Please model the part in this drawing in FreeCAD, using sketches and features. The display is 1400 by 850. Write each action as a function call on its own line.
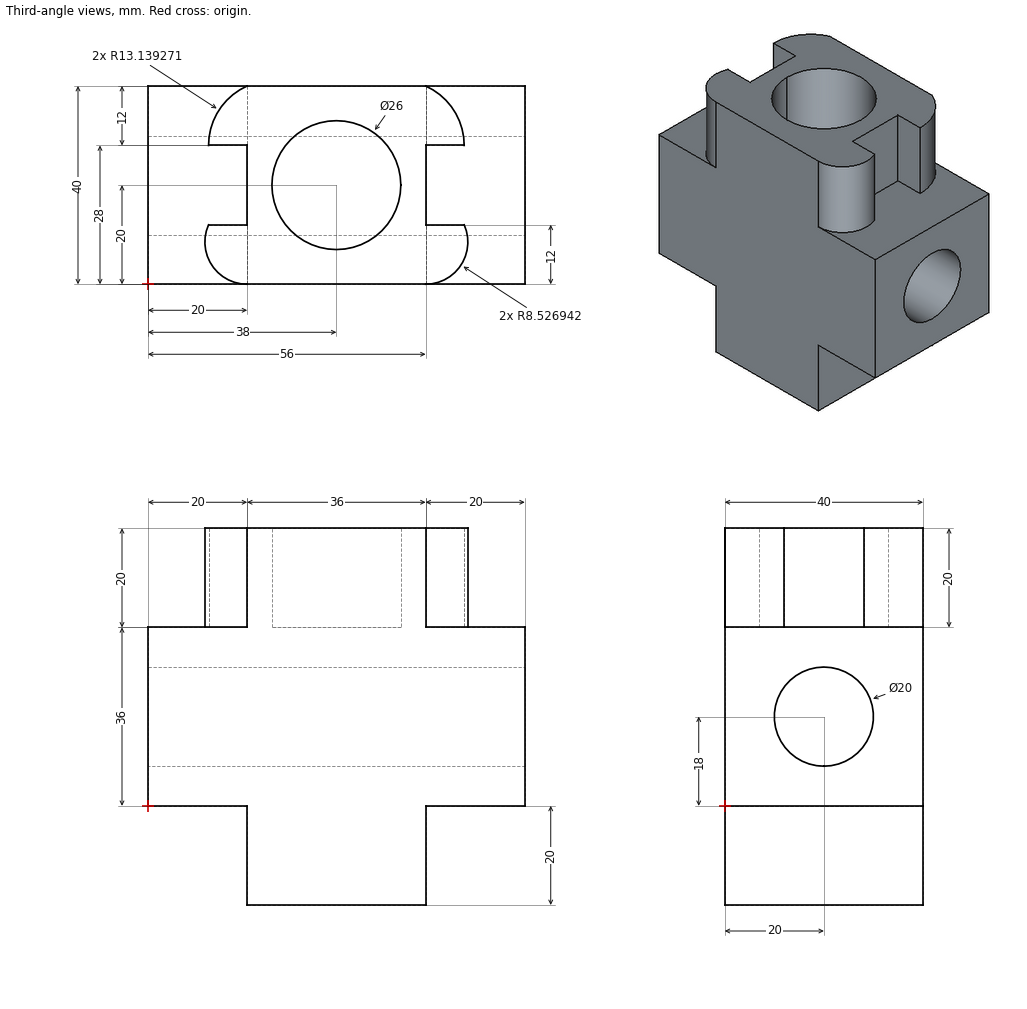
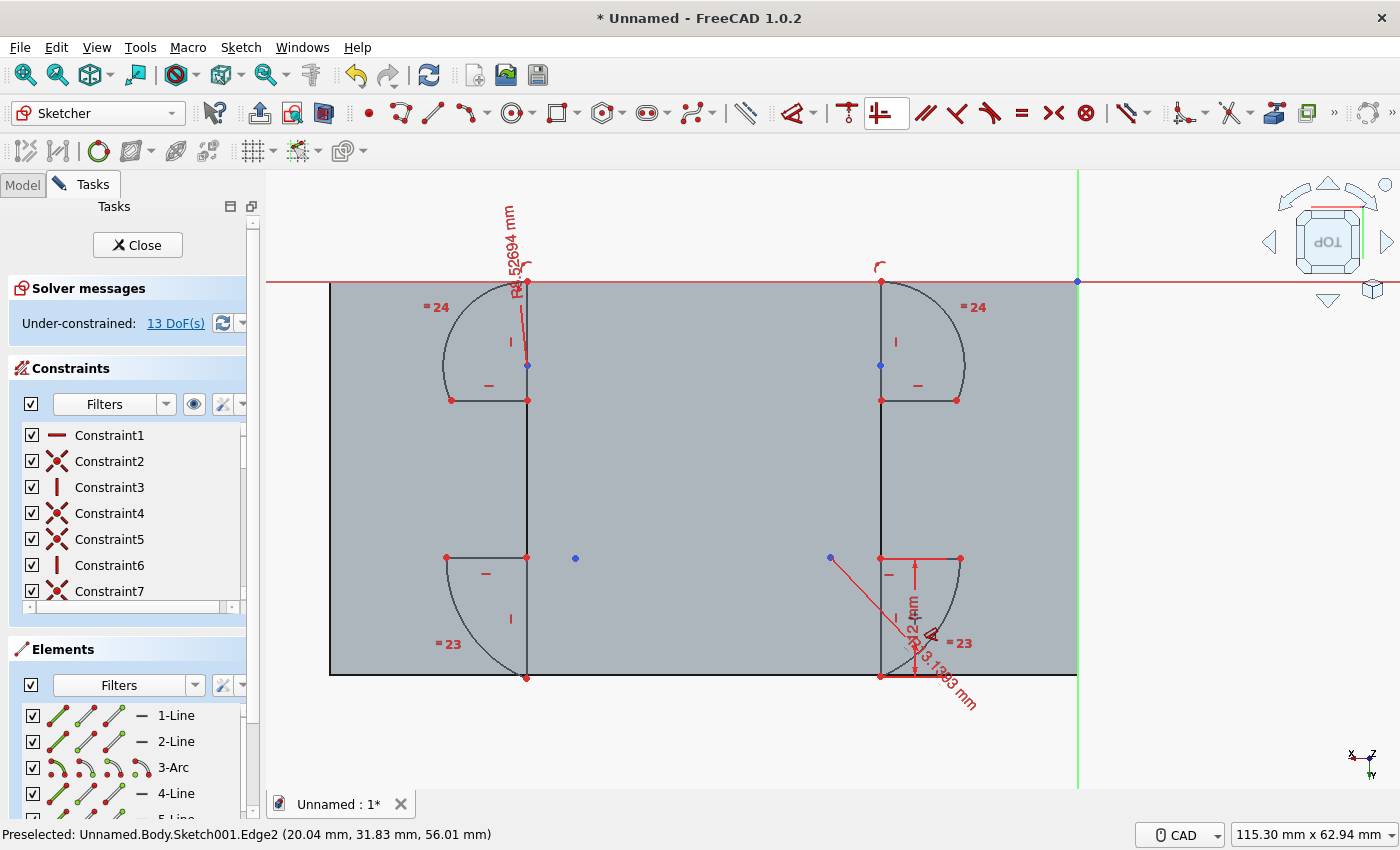
click(527, 642)
click(493, 618)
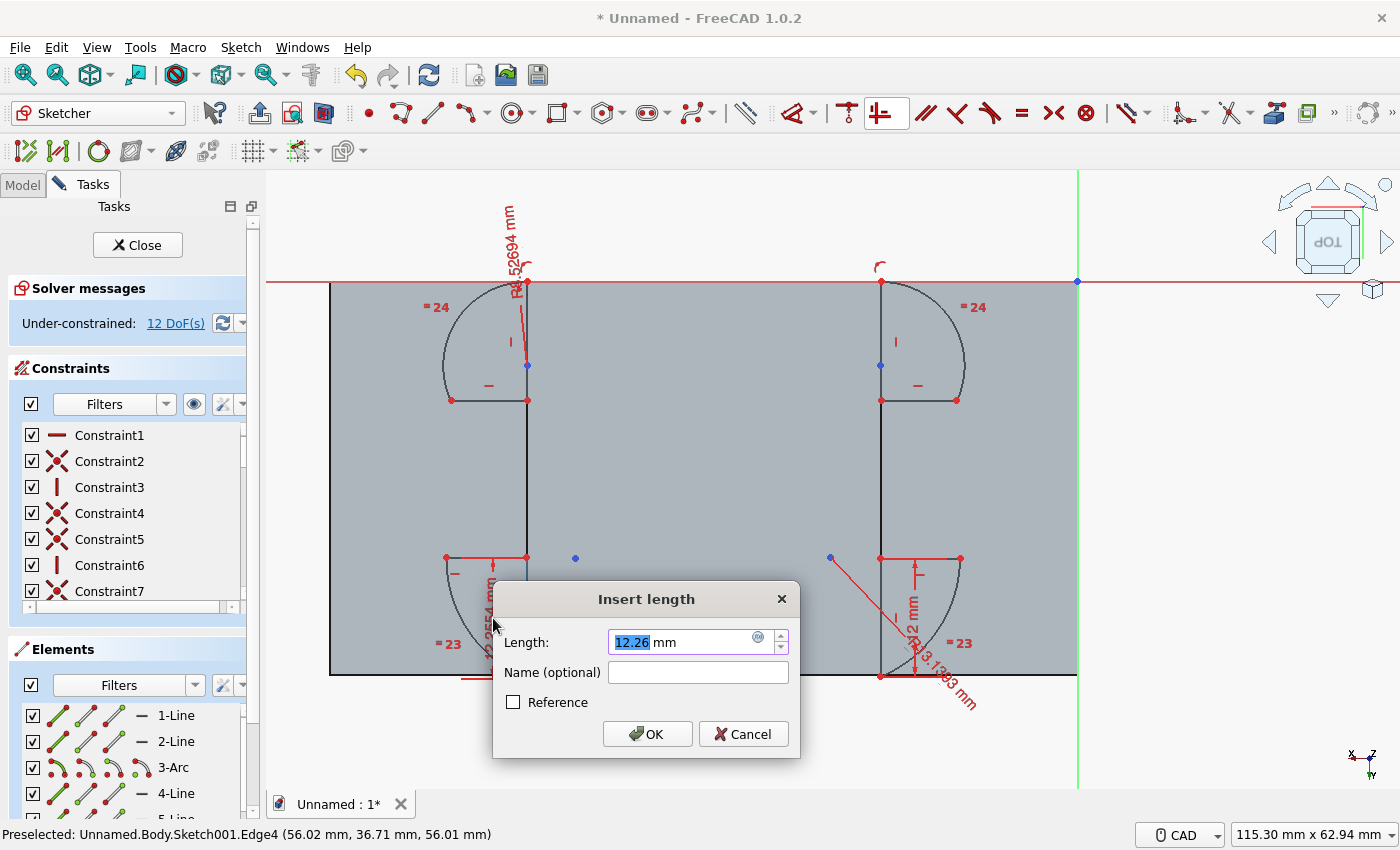
text(12)
key(Return)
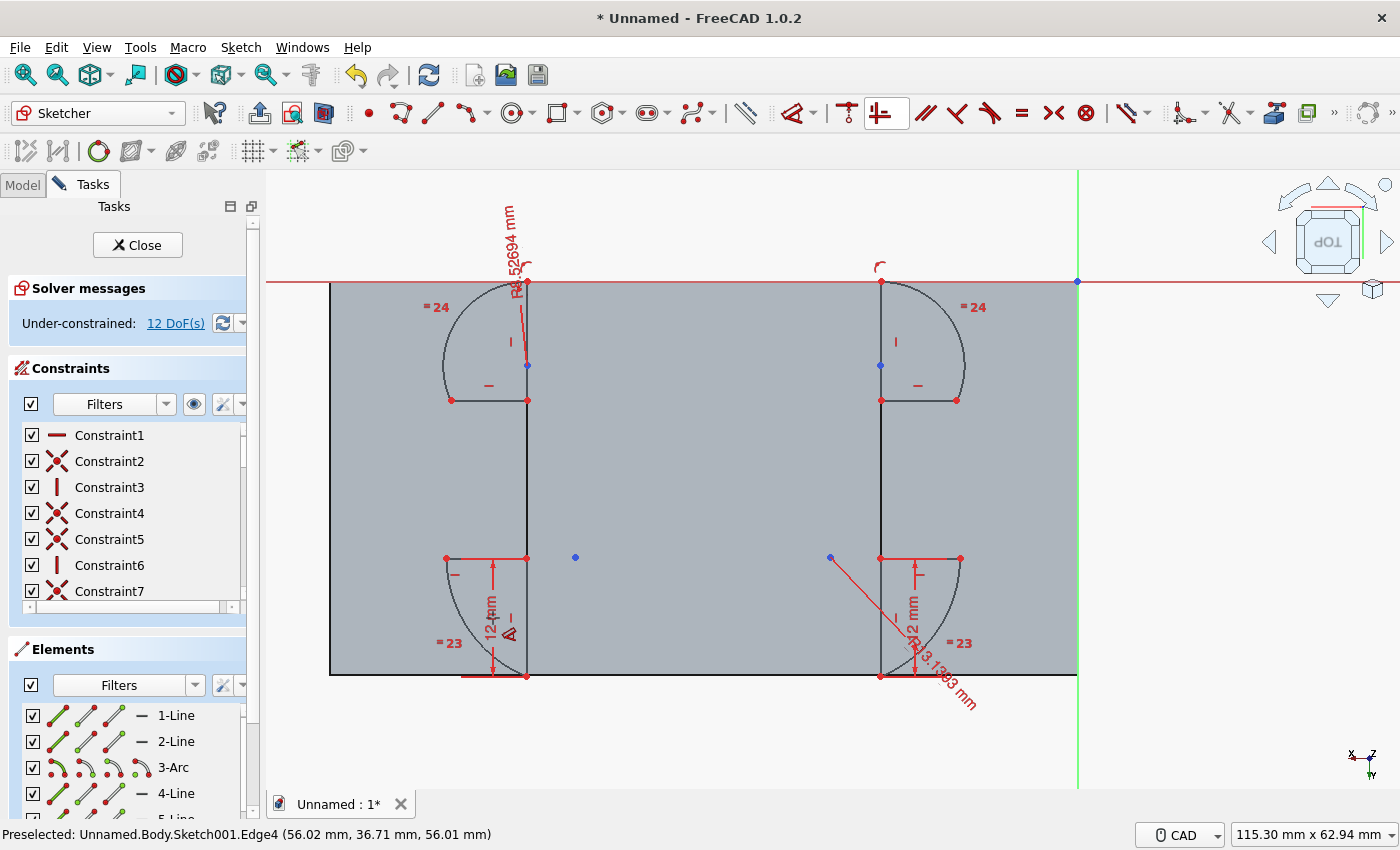
click(527, 318)
click(493, 341)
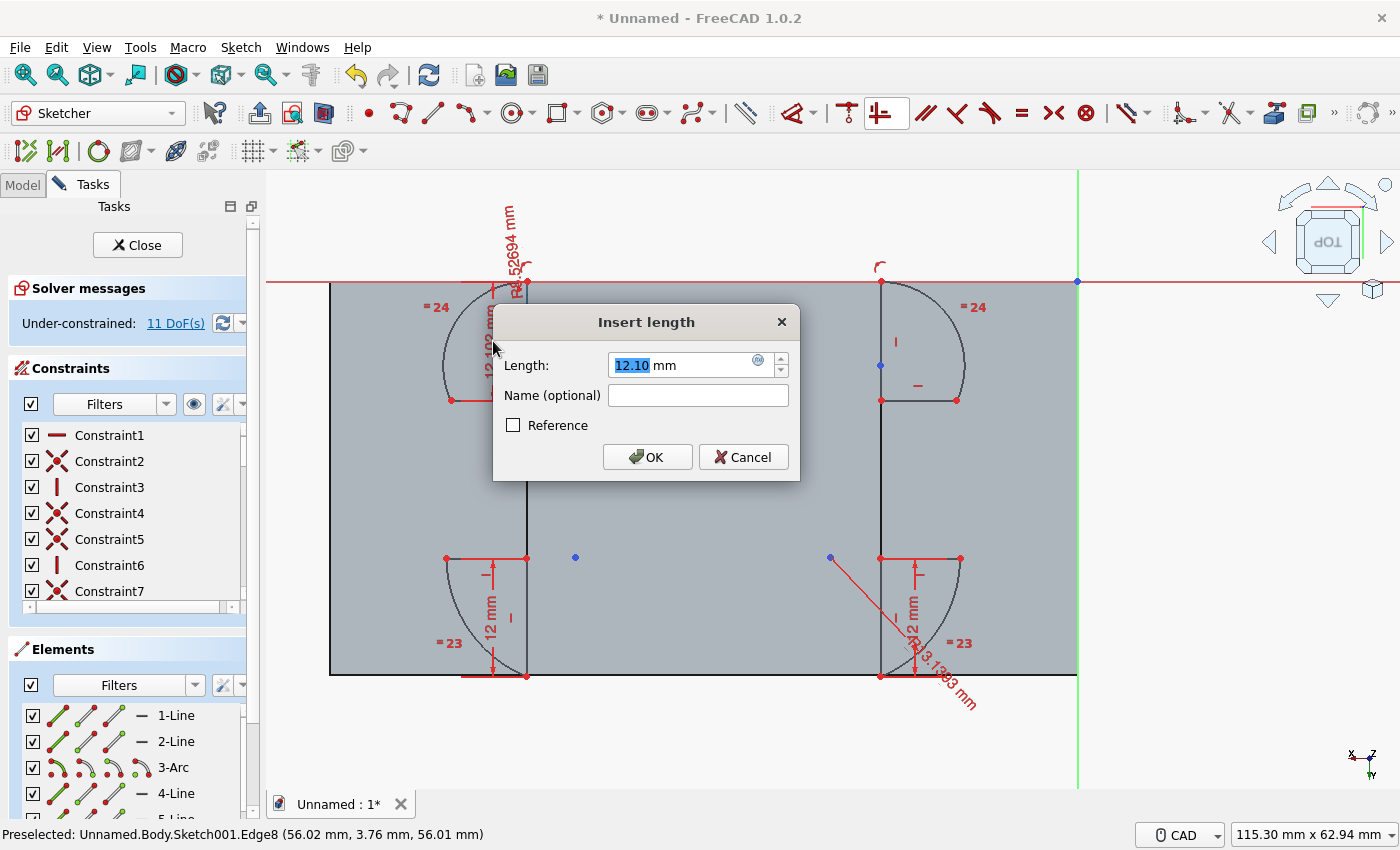
text(12)
key(Return)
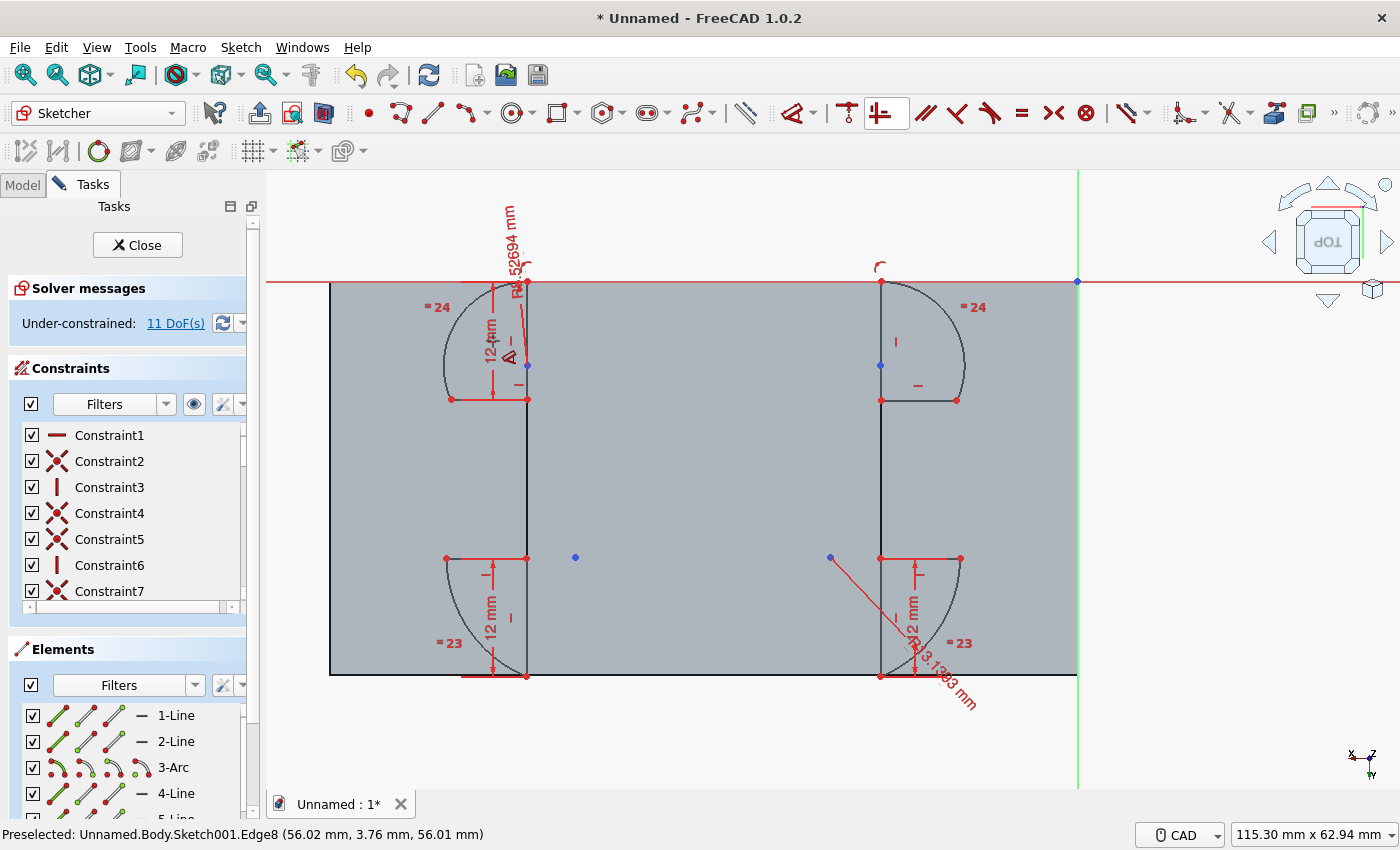
click(881, 318)
click(915, 341)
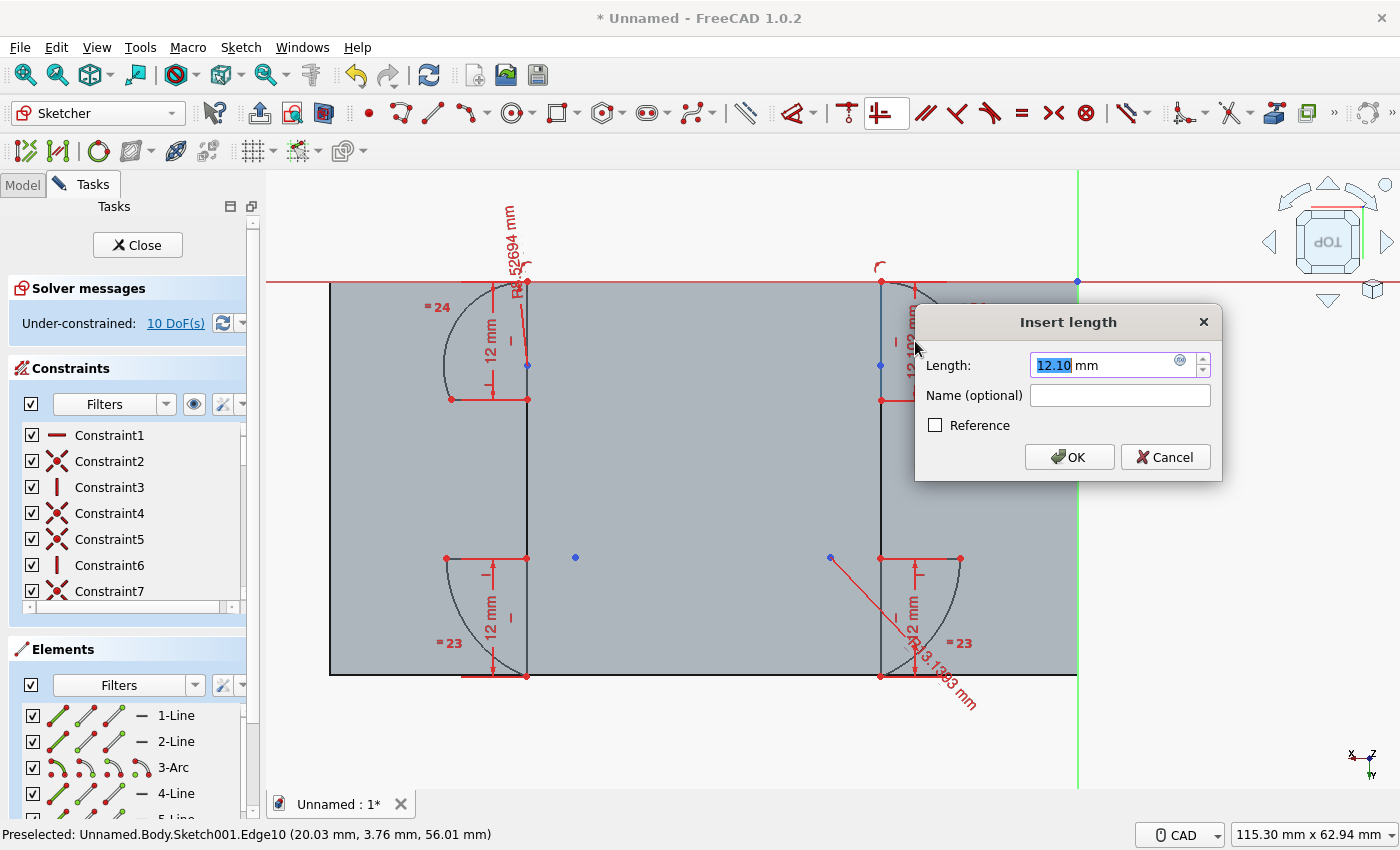
text(12)
key(Return)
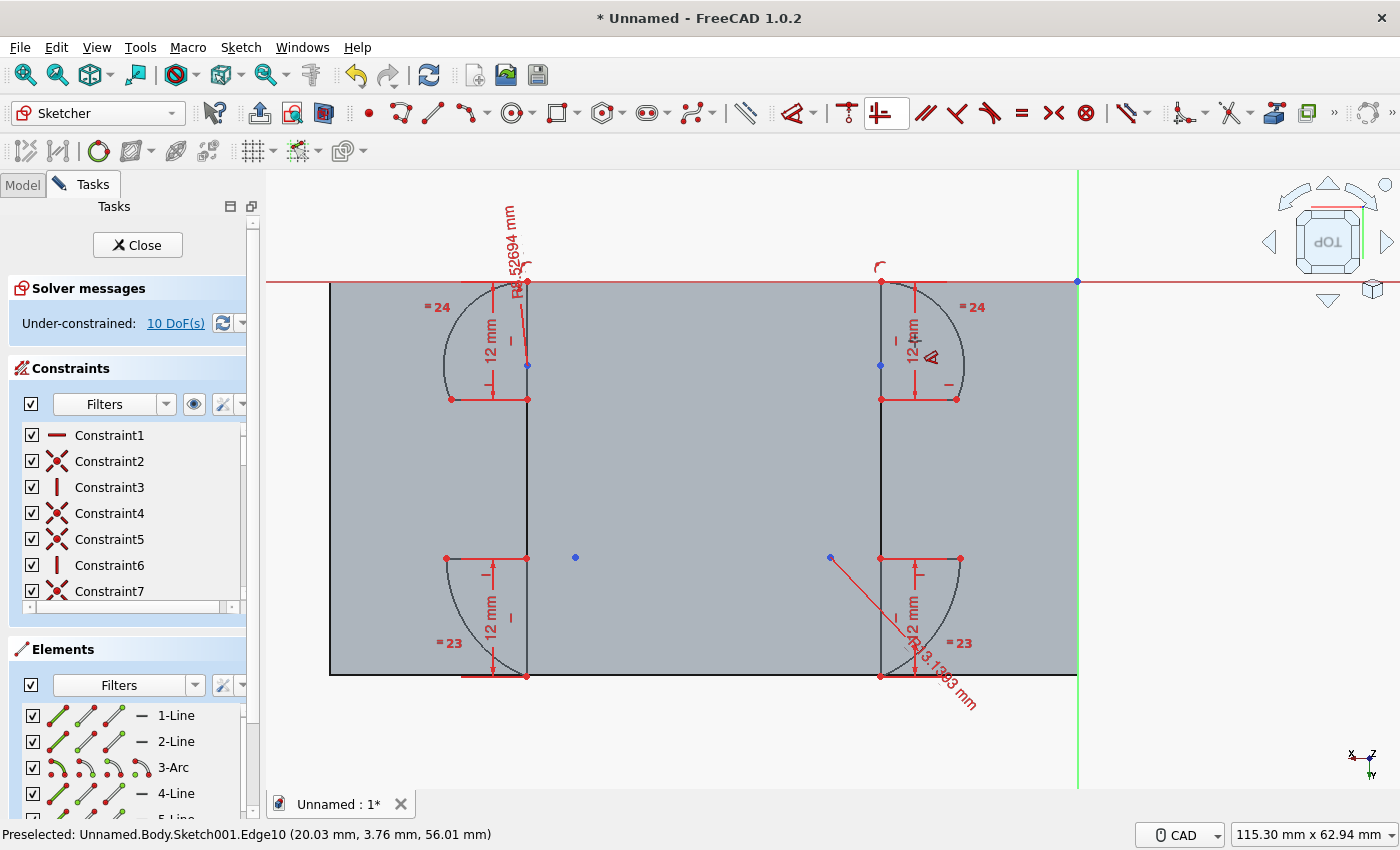
click(960, 559)
click(1112, 420)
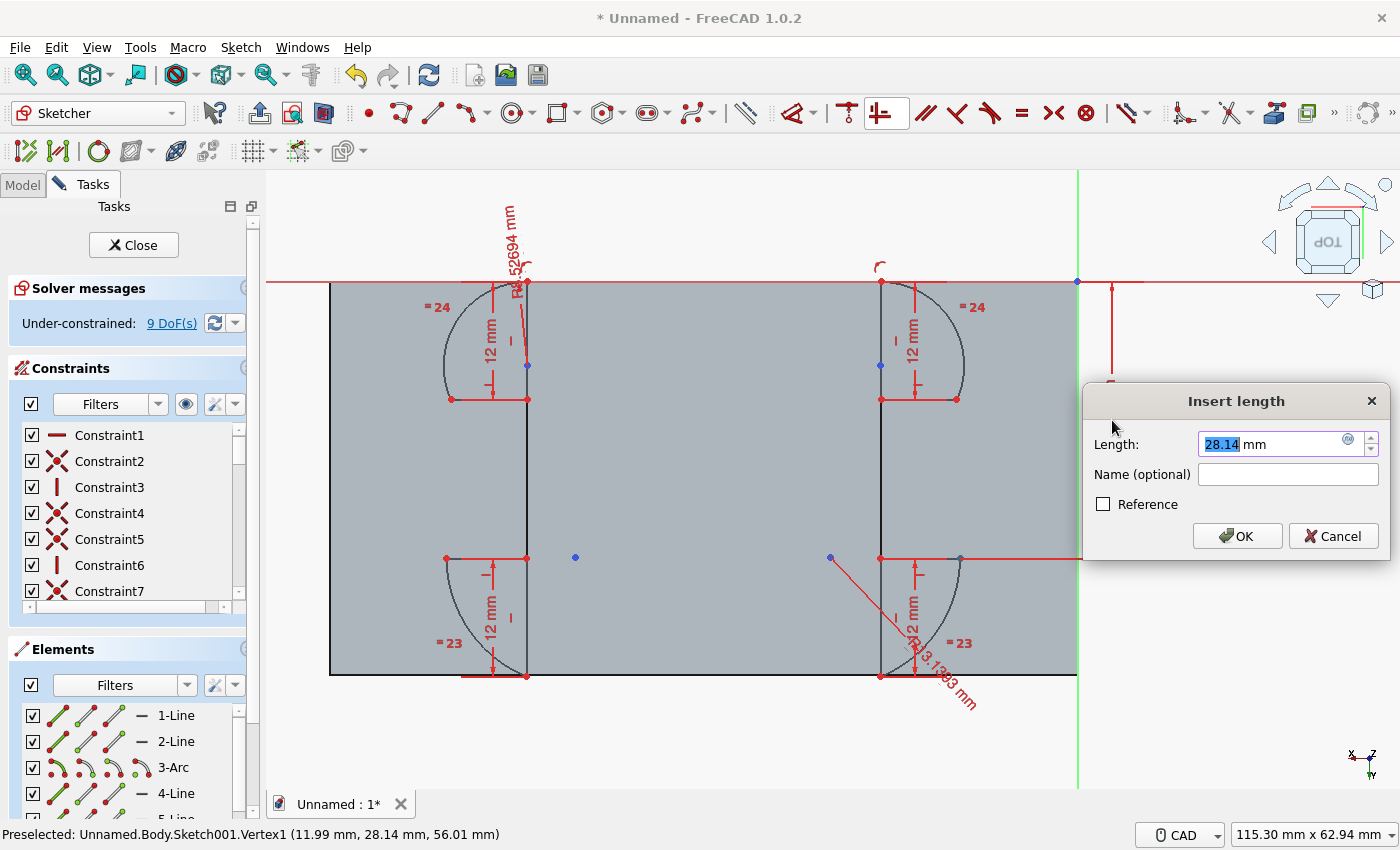
text(28)
key(Return)